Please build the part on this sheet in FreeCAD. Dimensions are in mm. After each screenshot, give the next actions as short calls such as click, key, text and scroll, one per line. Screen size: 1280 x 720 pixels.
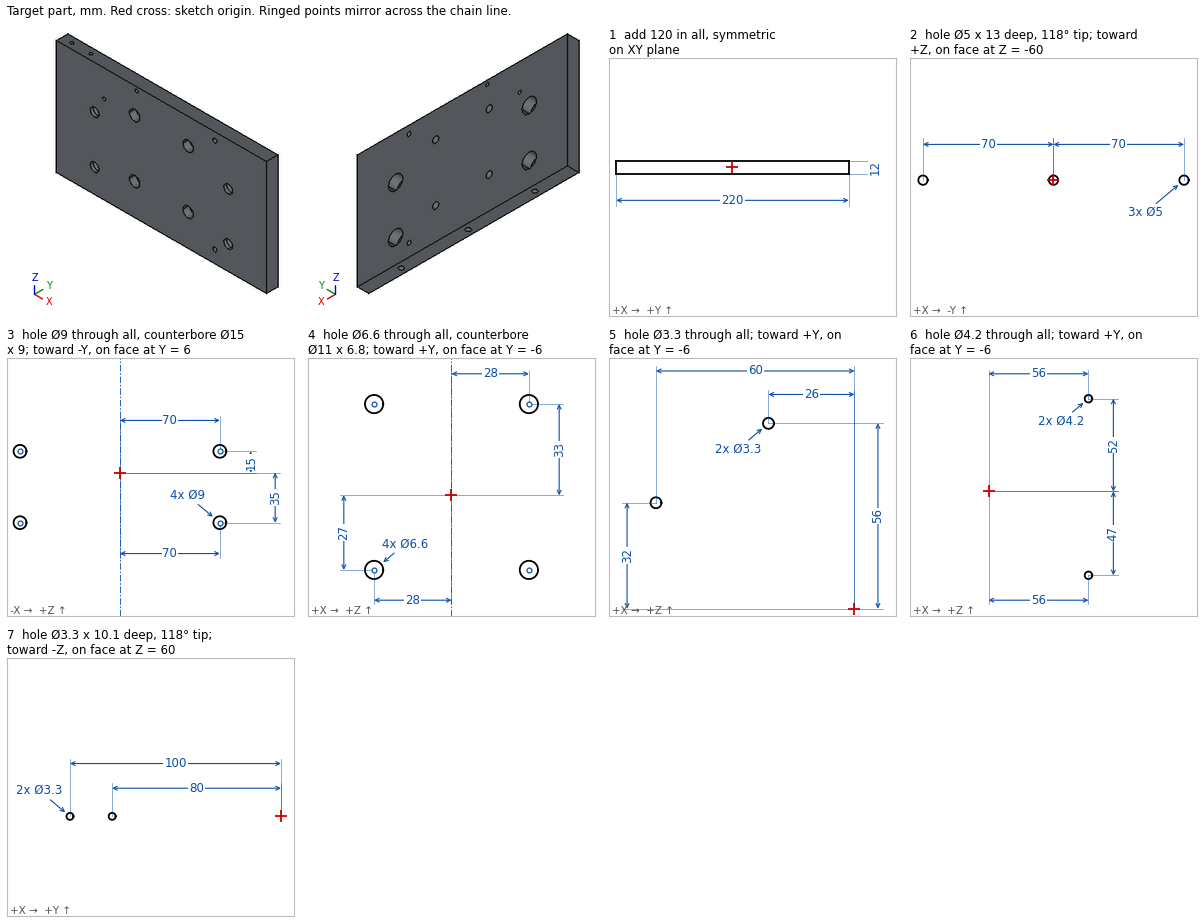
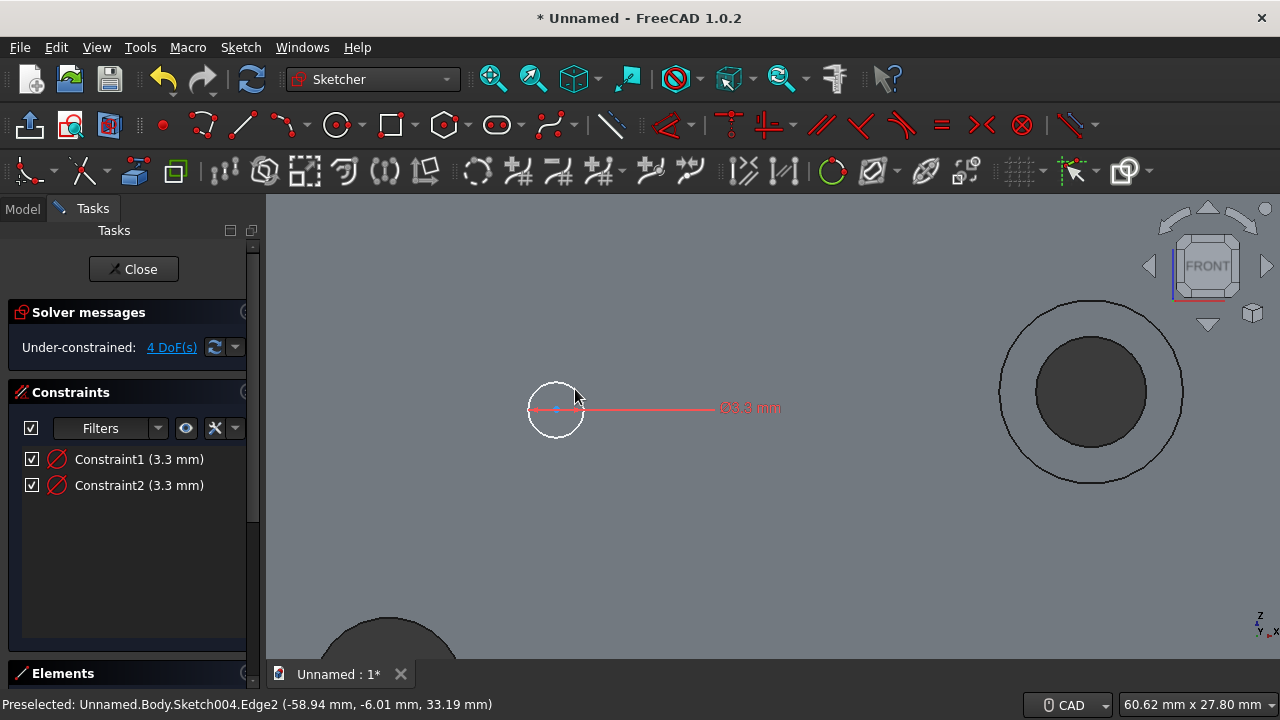
click(666, 126)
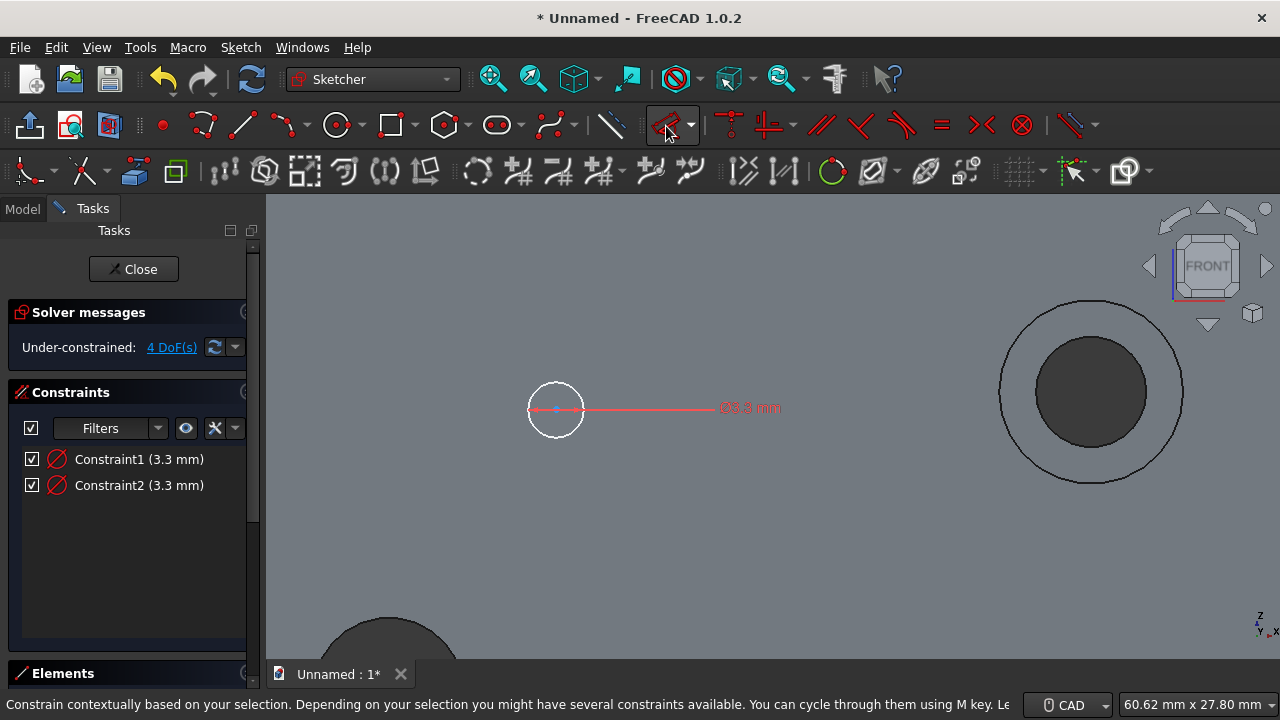
scroll(558, 411, down, 6)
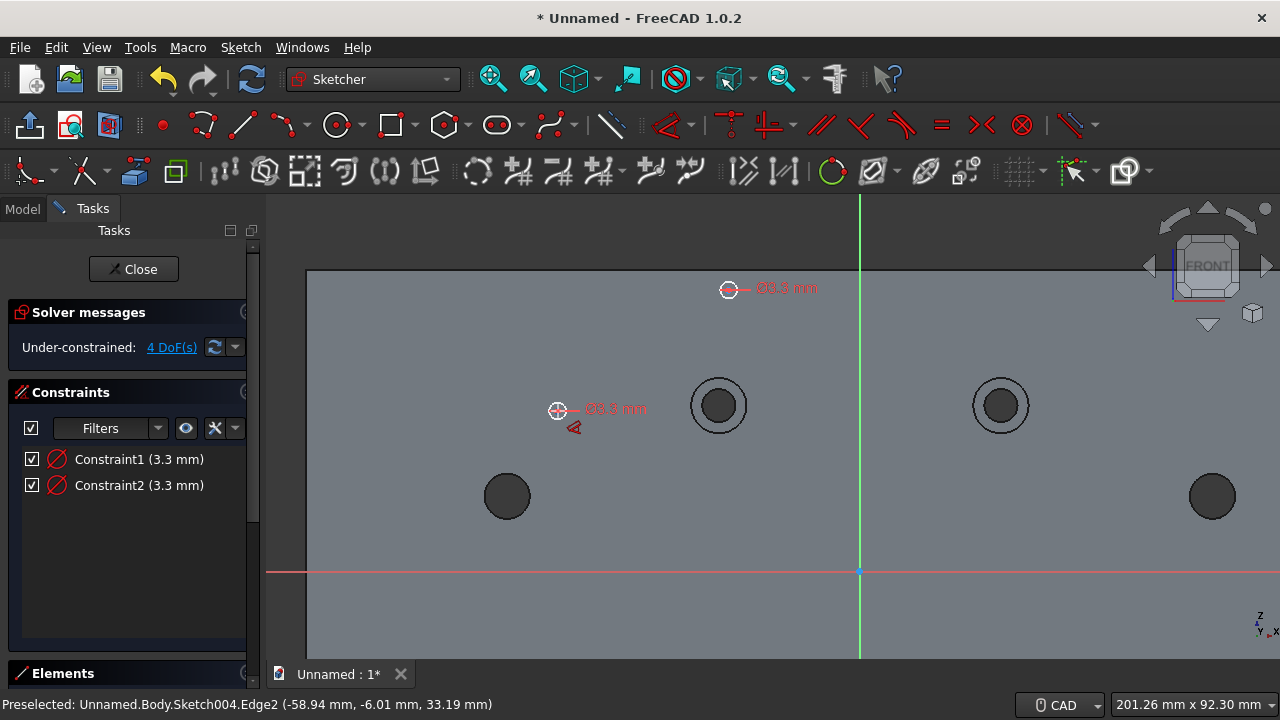
click(729, 290)
click(794, 606)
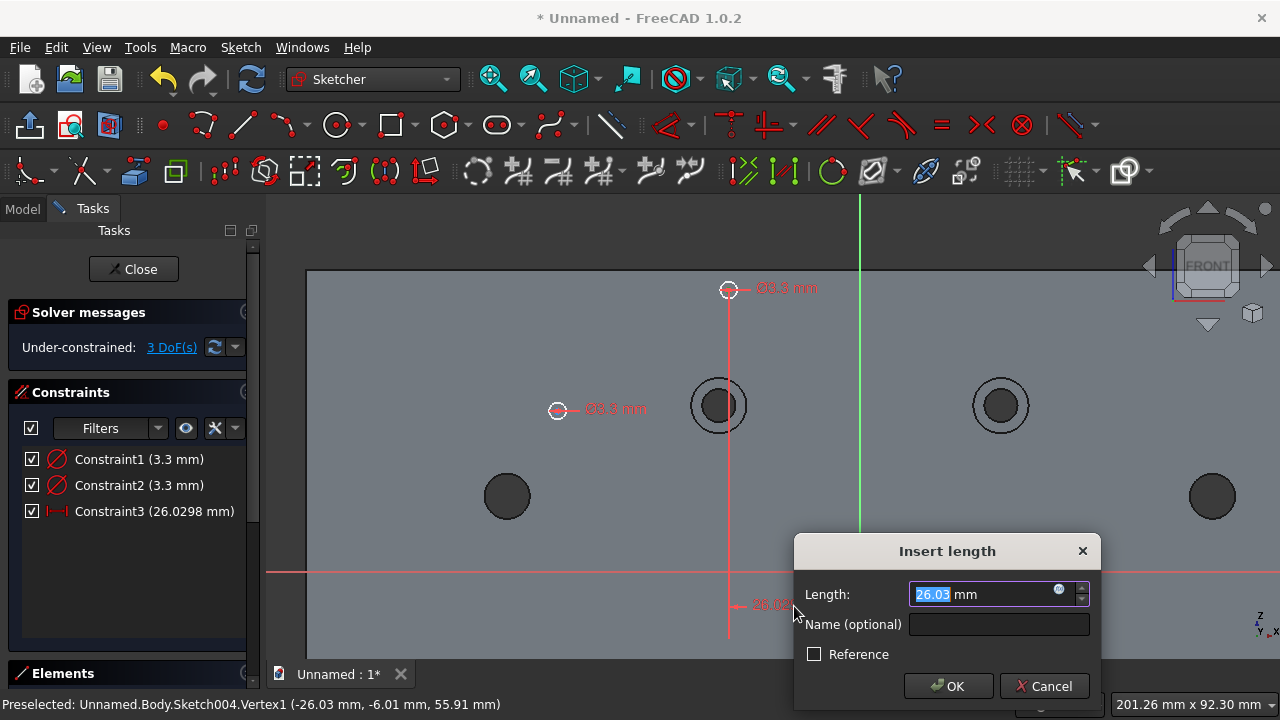
text(26)
key(Return)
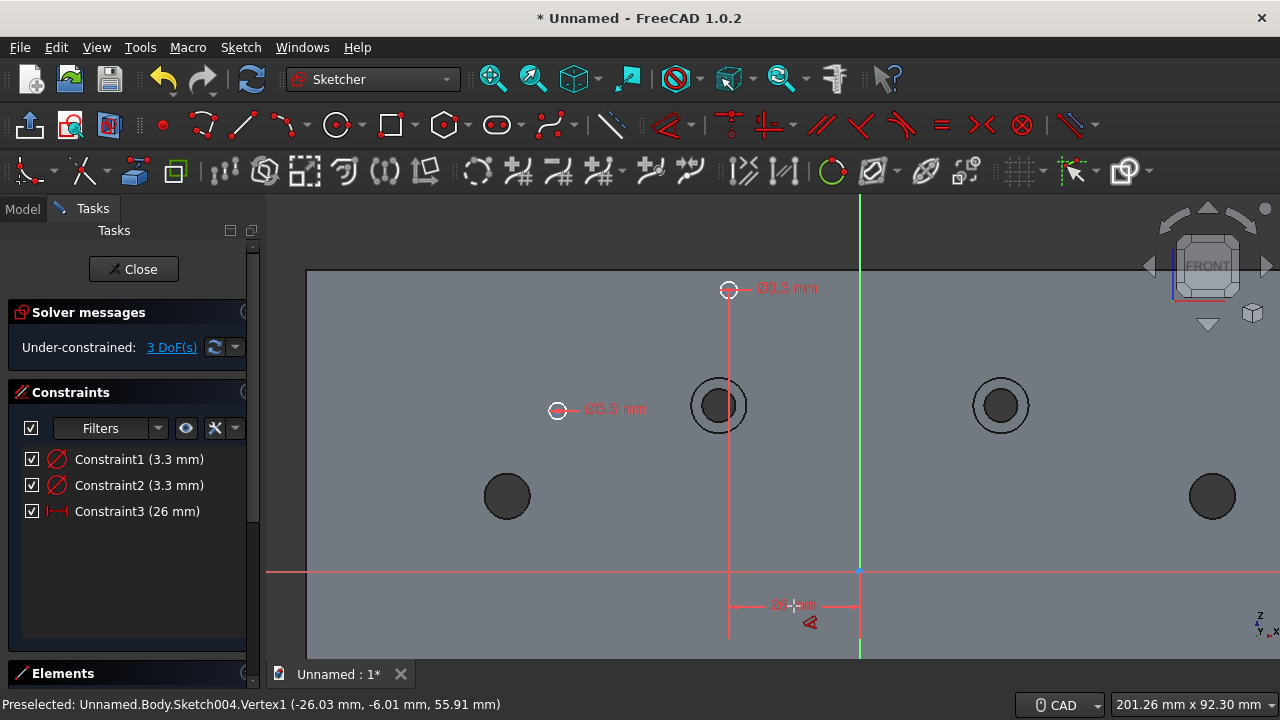
click(729, 290)
click(894, 431)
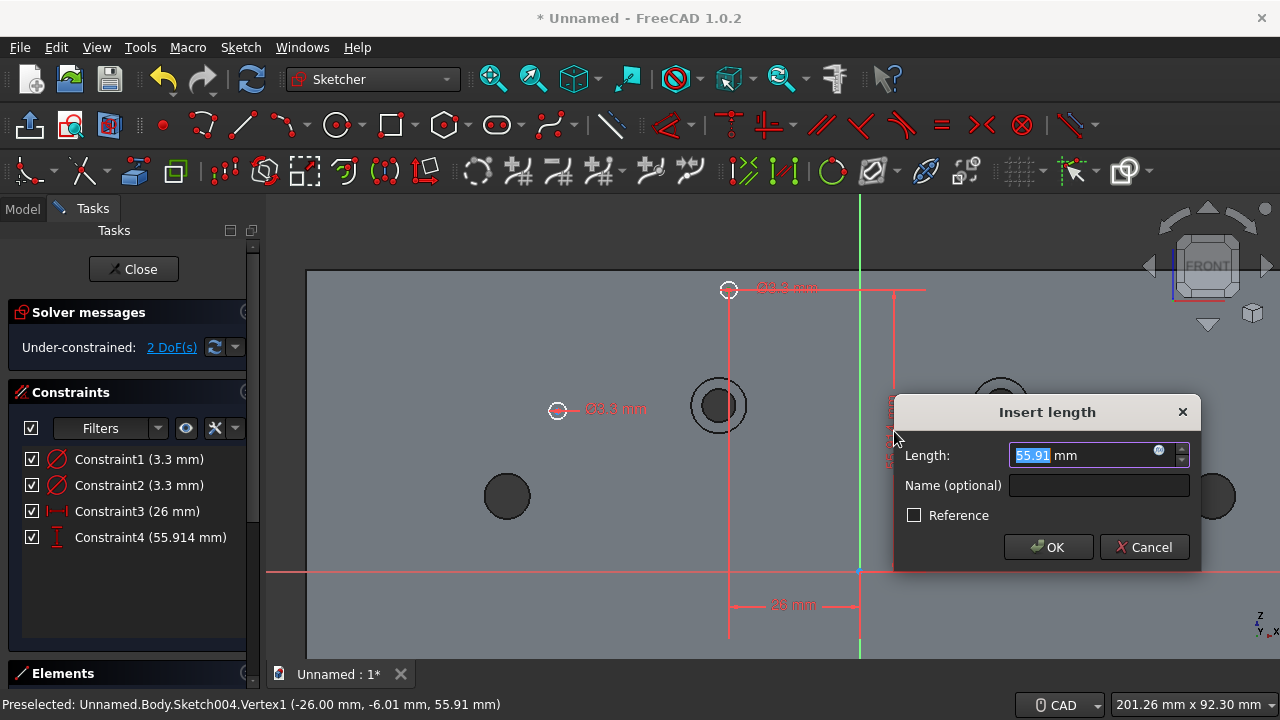
text(56)
key(Return)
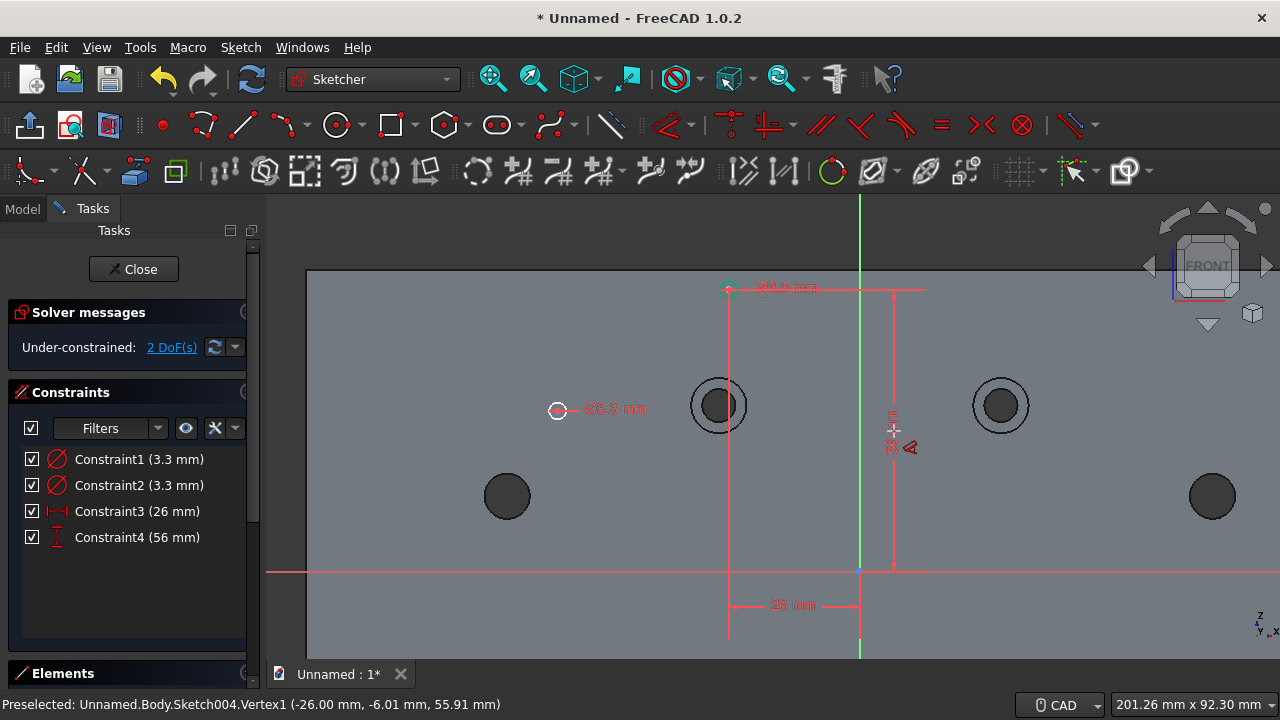
click(558, 411)
click(709, 606)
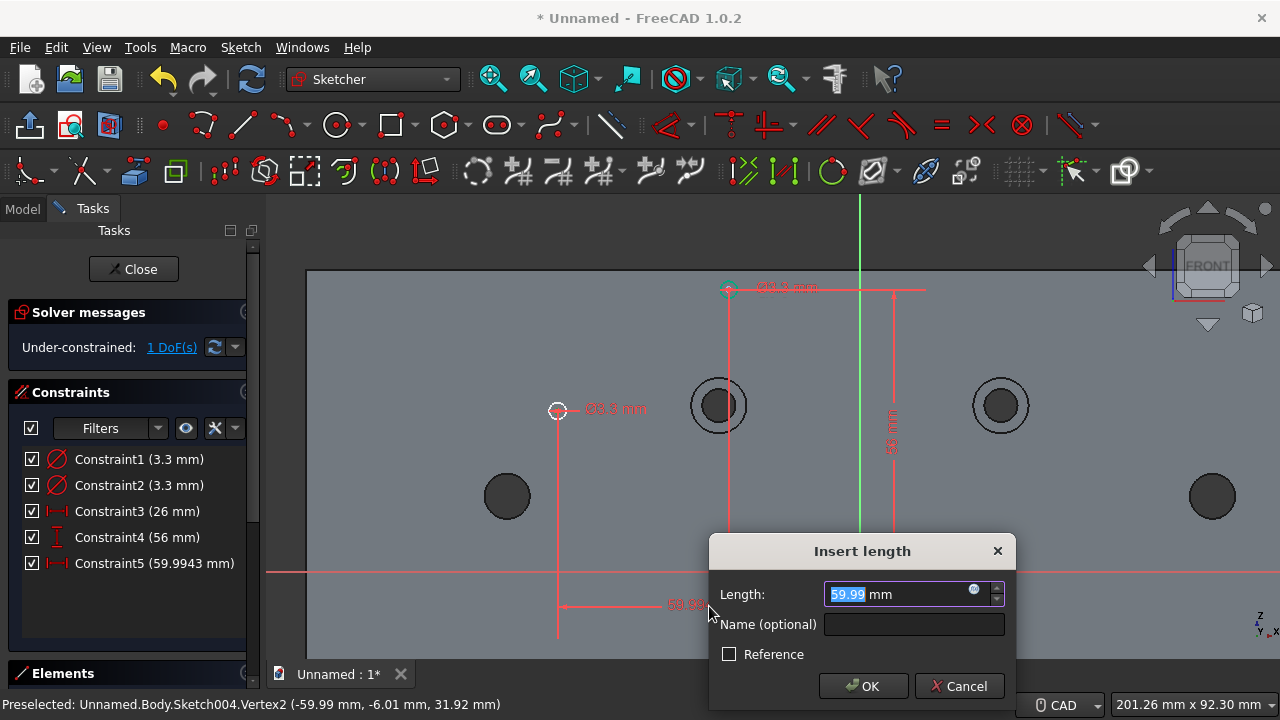
text(60)
key(Return)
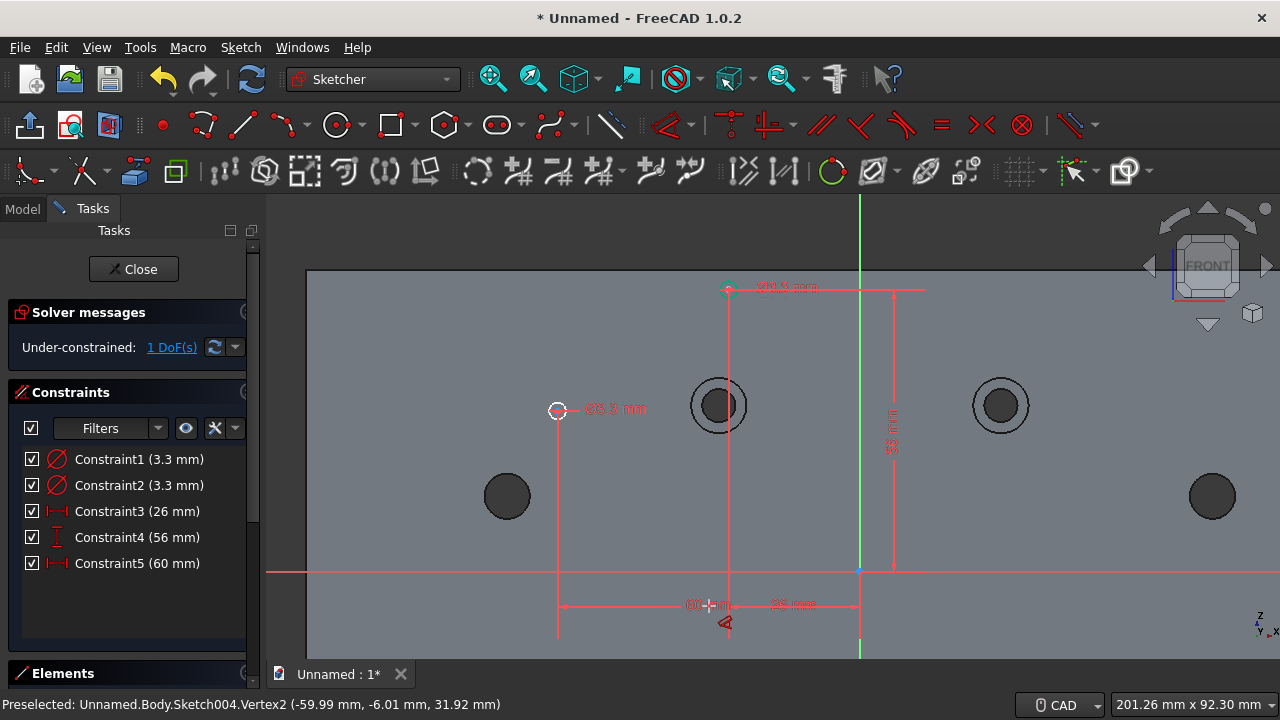
click(558, 411)
click(894, 491)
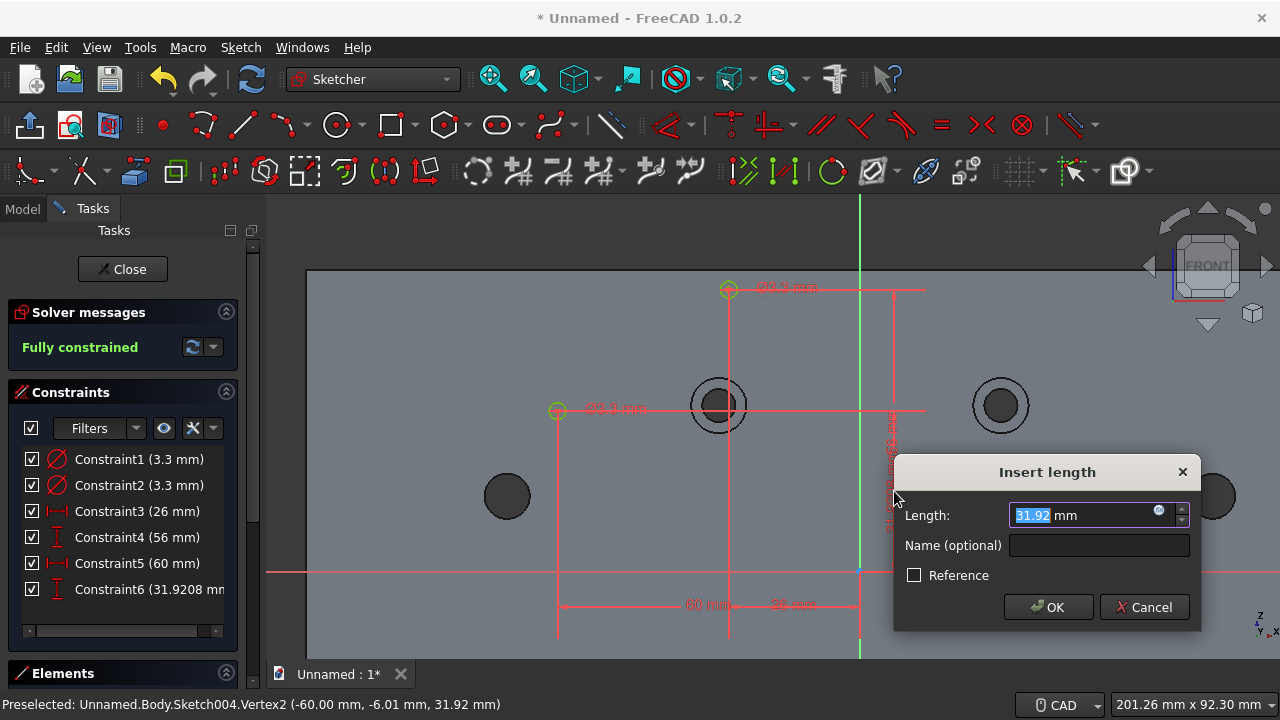
text(32)
key(Return)
key(Escape)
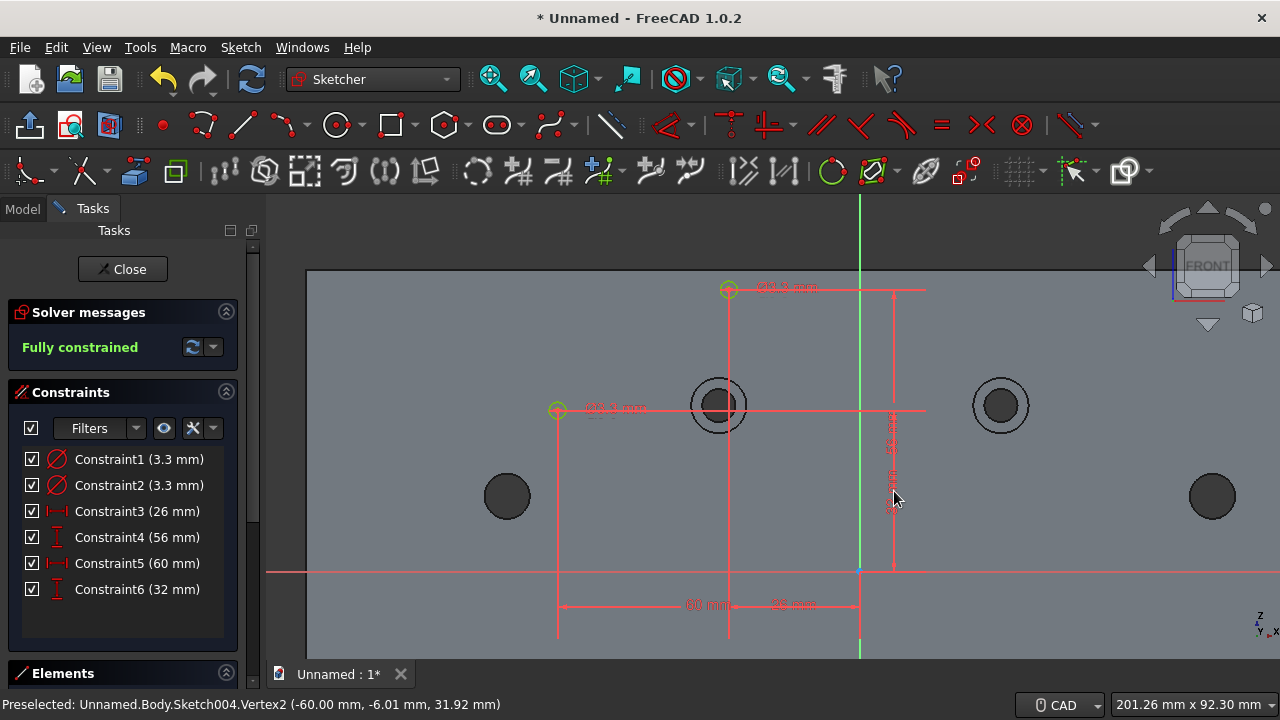
click(123, 269)